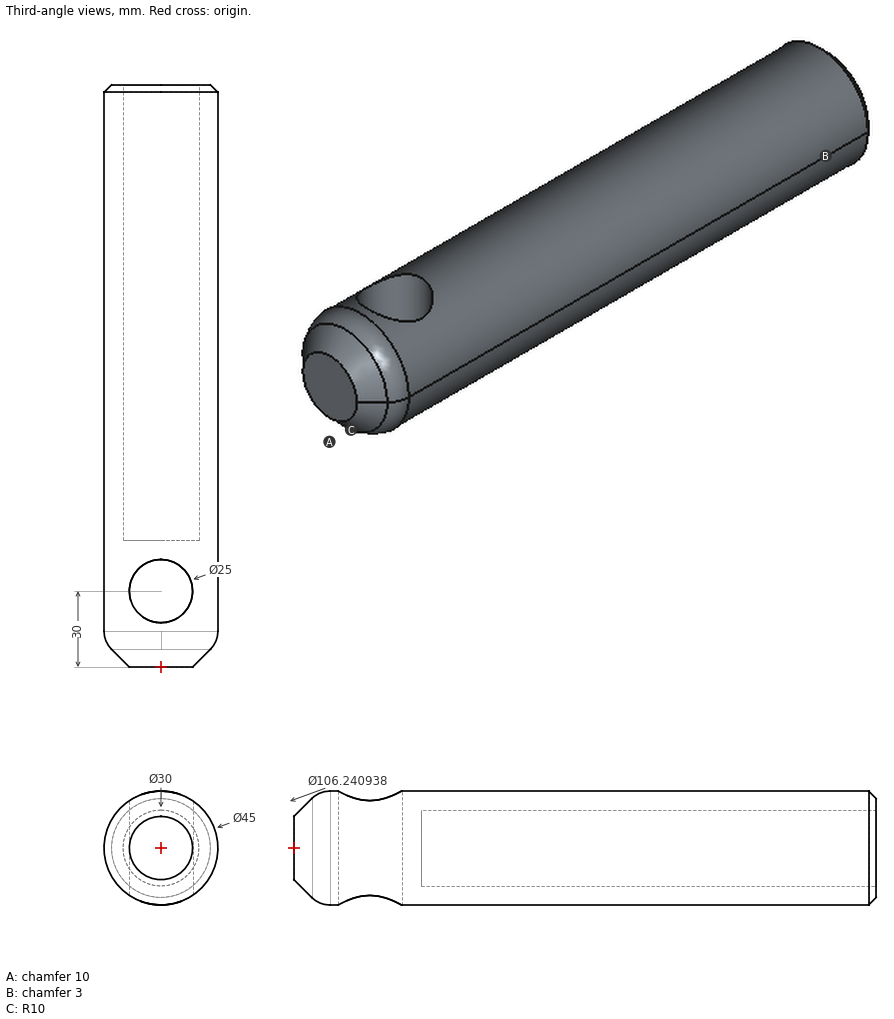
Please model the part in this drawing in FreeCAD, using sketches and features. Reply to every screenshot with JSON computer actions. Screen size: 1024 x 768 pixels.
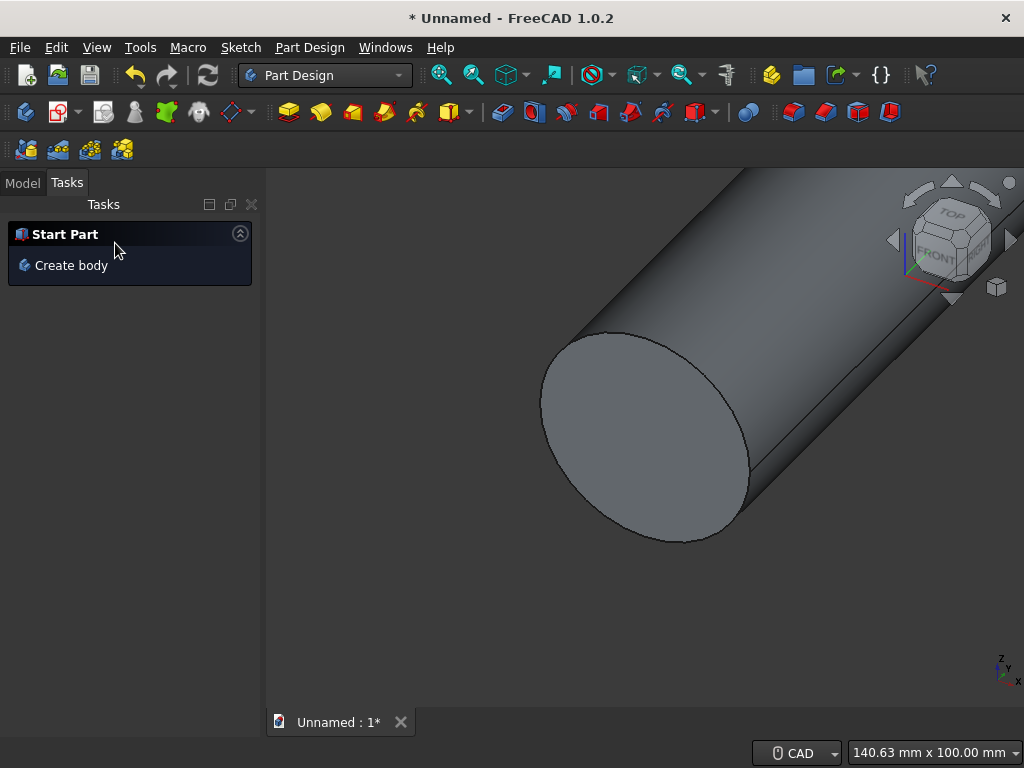
{"action": "key", "text": "v f"}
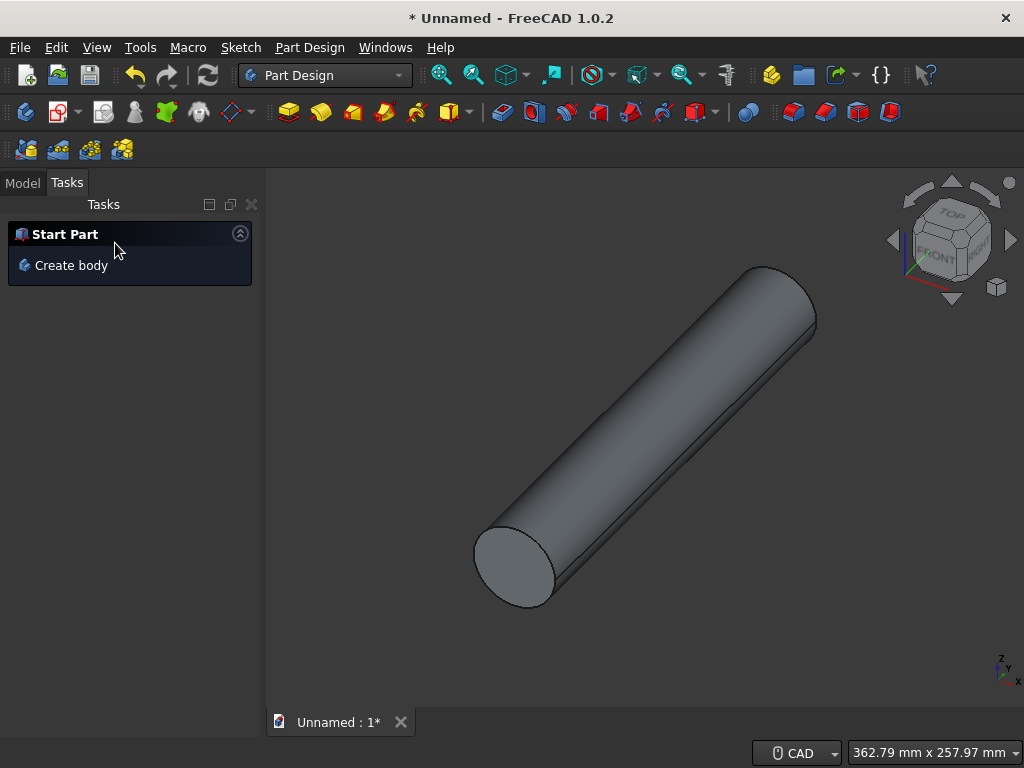
{"action": "key", "text": "4"}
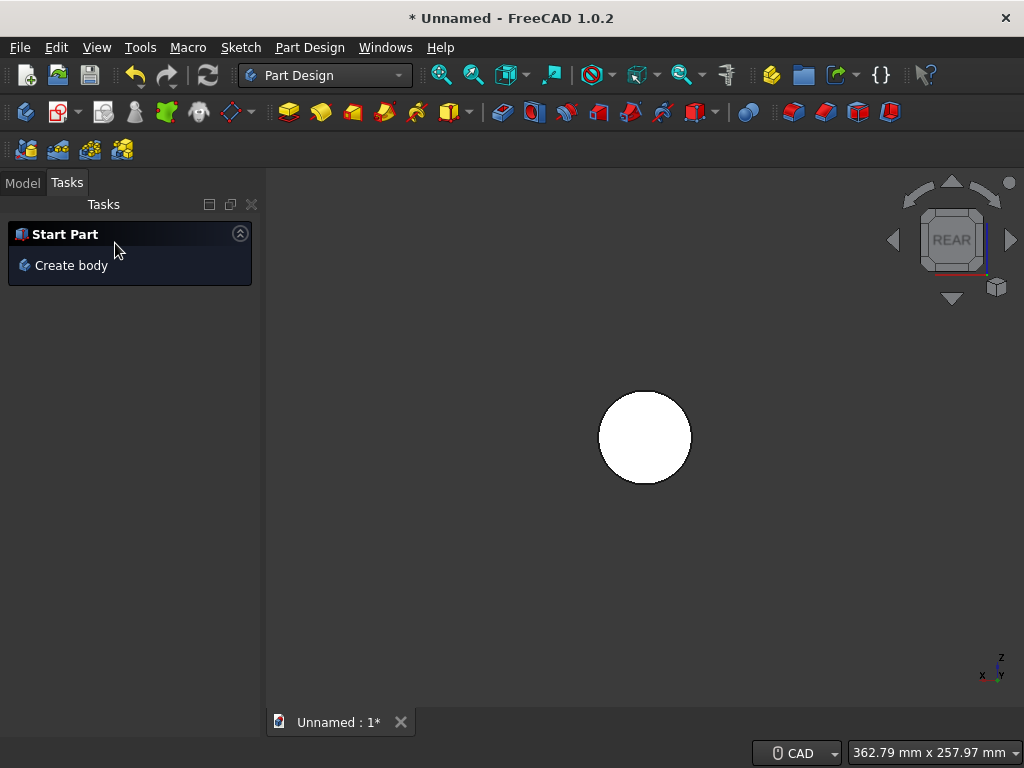
{"action": "left_click", "coordinate": [442, 76]}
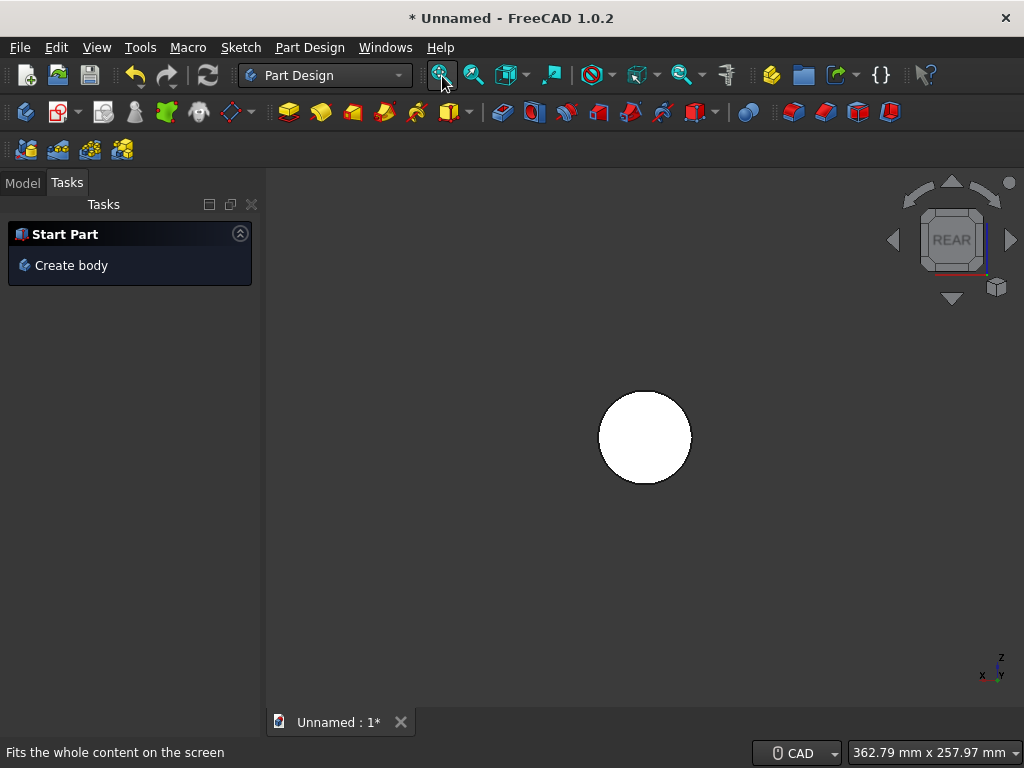
{"action": "left_click", "coordinate": [645, 437]}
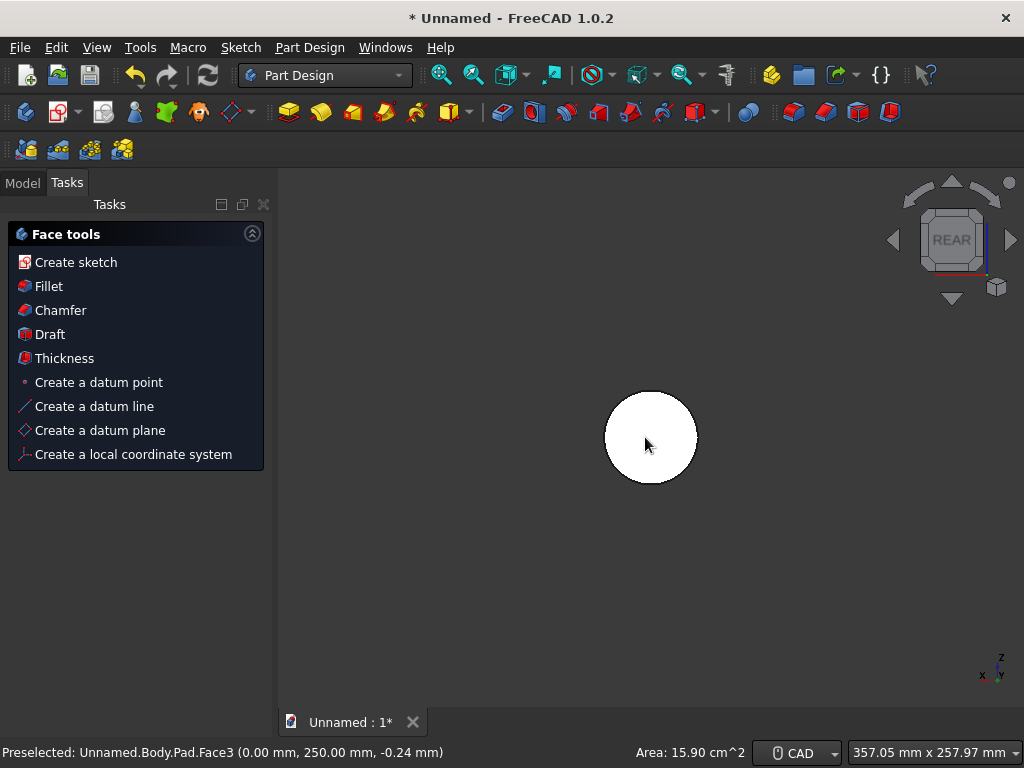
{"action": "left_click", "coordinate": [58, 112]}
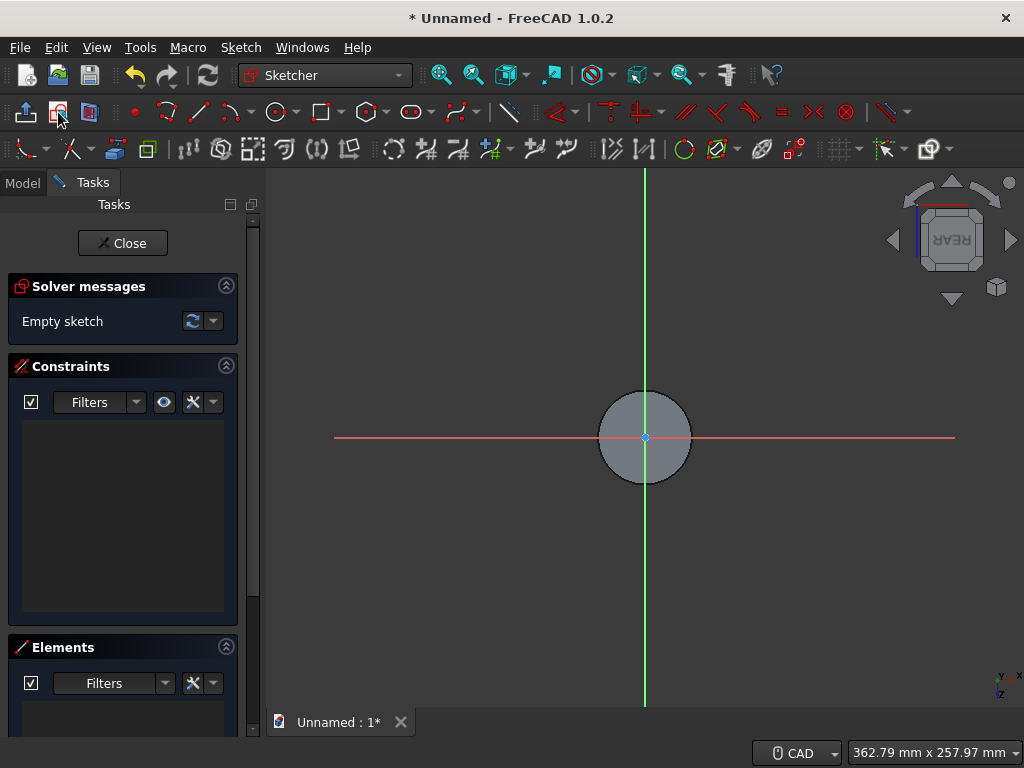
{"action": "scroll", "coordinate": [662, 437], "scroll_direction": "up", "scroll_amount": 8}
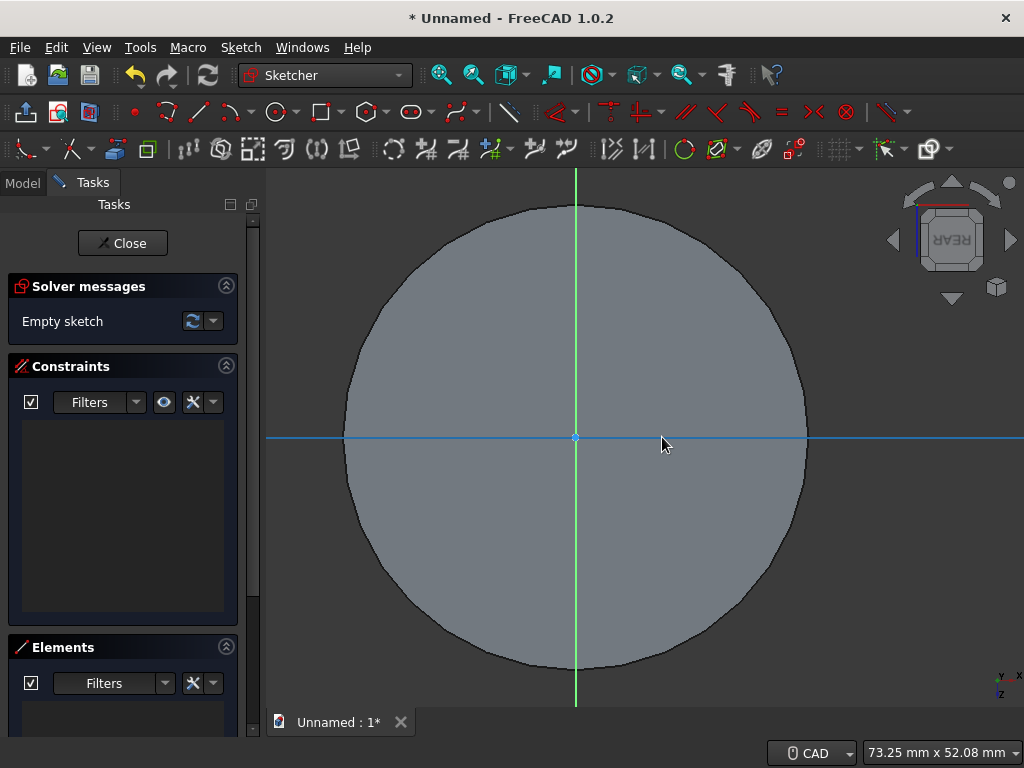
{"action": "left_click", "coordinate": [276, 112]}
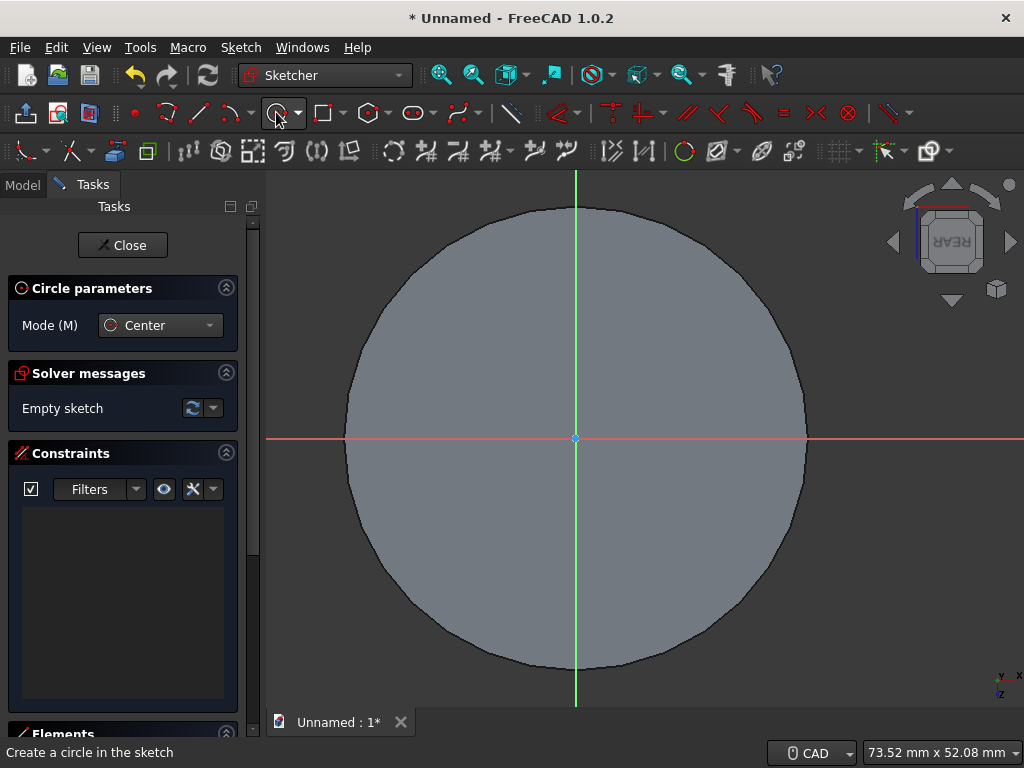
{"action": "left_click", "coordinate": [576, 438]}
{"action": "mouse_move", "coordinate": [685, 329]}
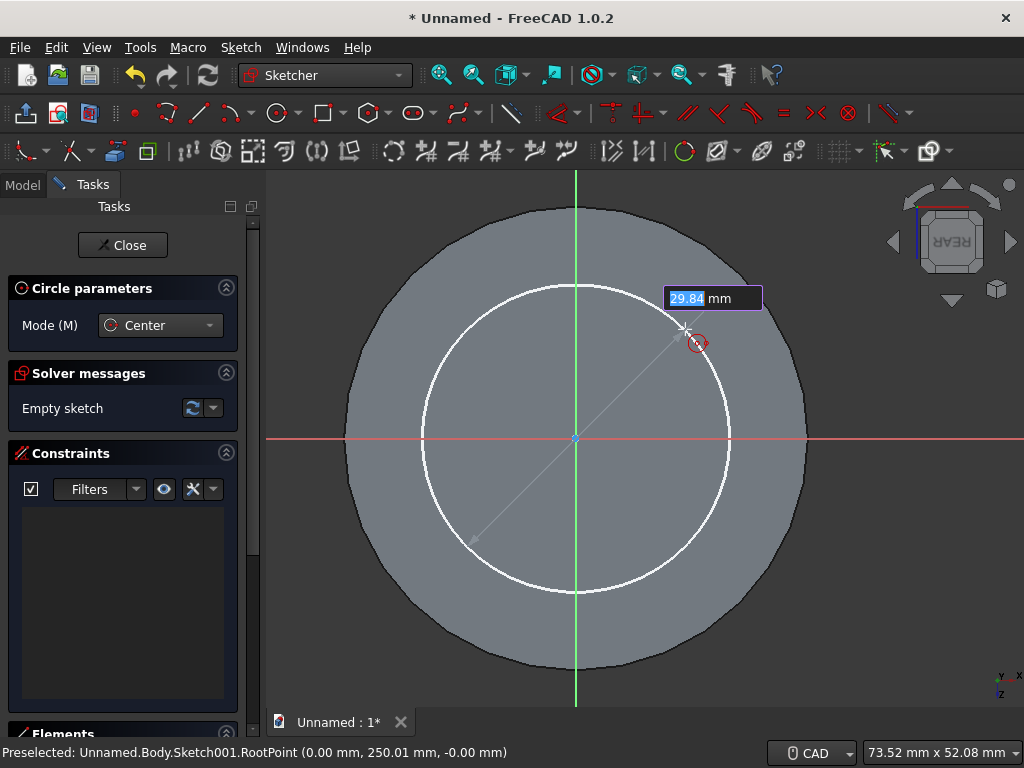
{"action": "type", "text": "30"}
{"action": "key", "text": "Return"}
{"action": "key", "text": "Escape"}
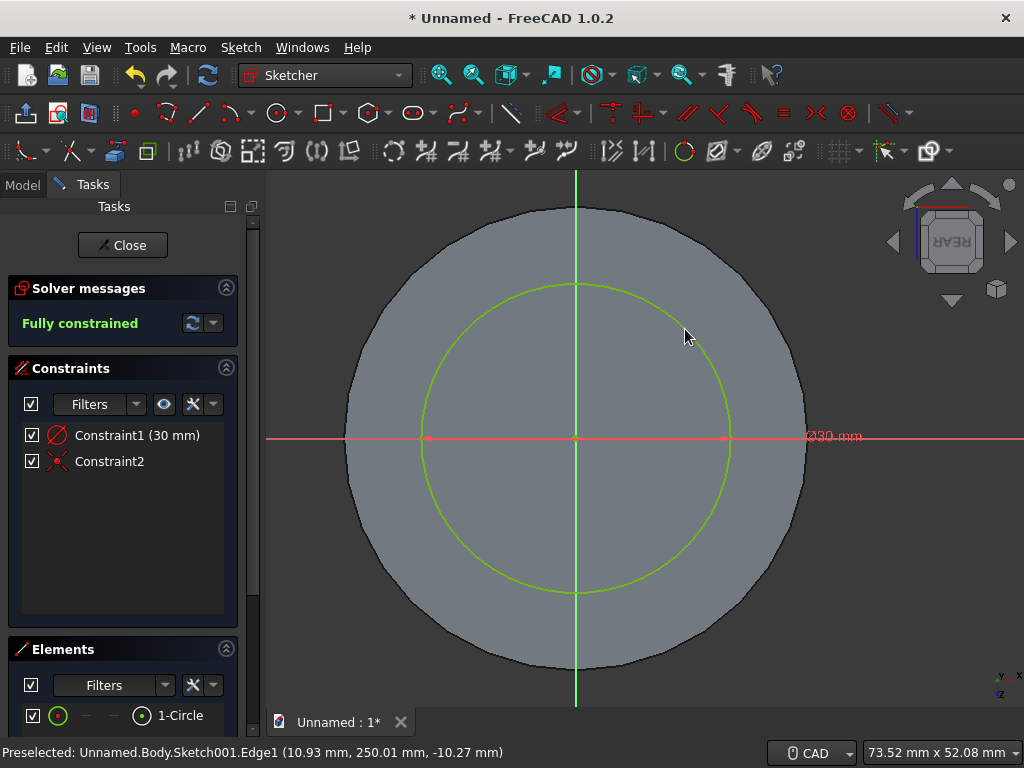
{"action": "left_click", "coordinate": [123, 245]}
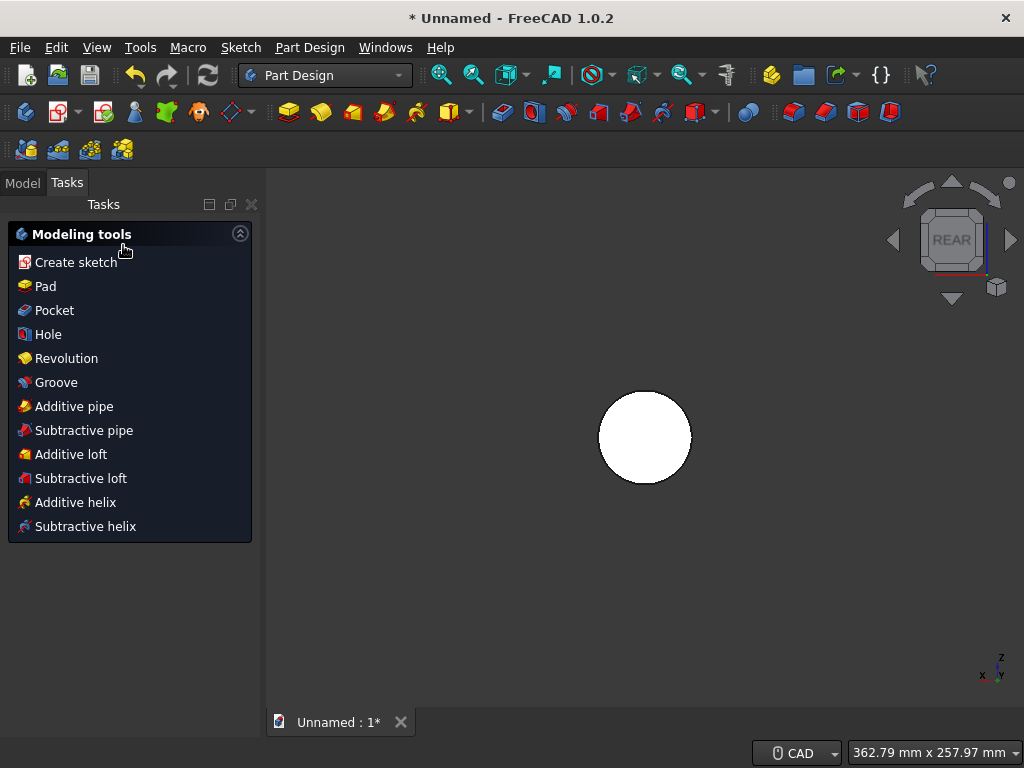
{"action": "left_click", "coordinate": [504, 112]}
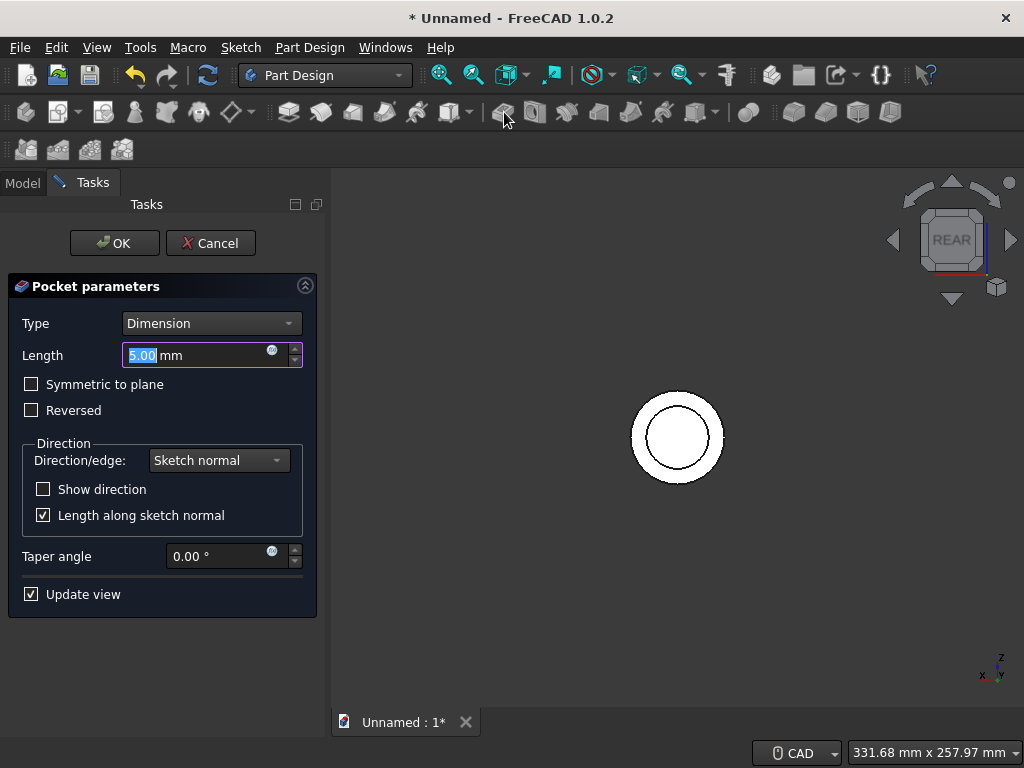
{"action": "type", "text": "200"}
{"action": "key", "text": "Tab"}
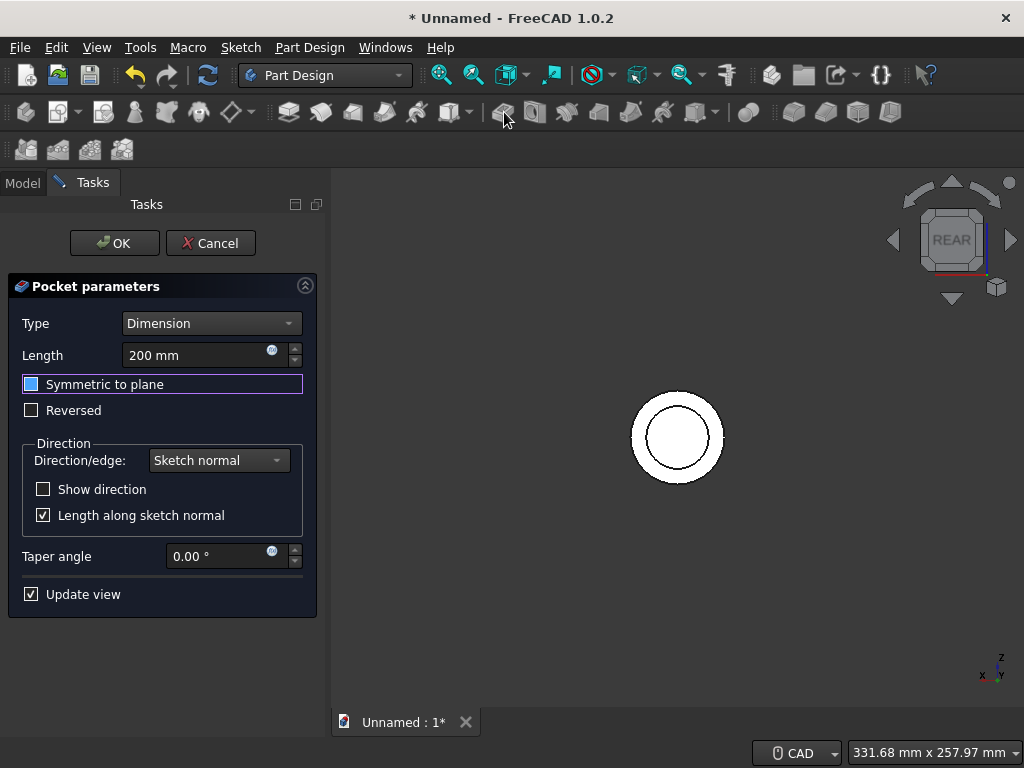
{"action": "left_click", "coordinate": [115, 243]}